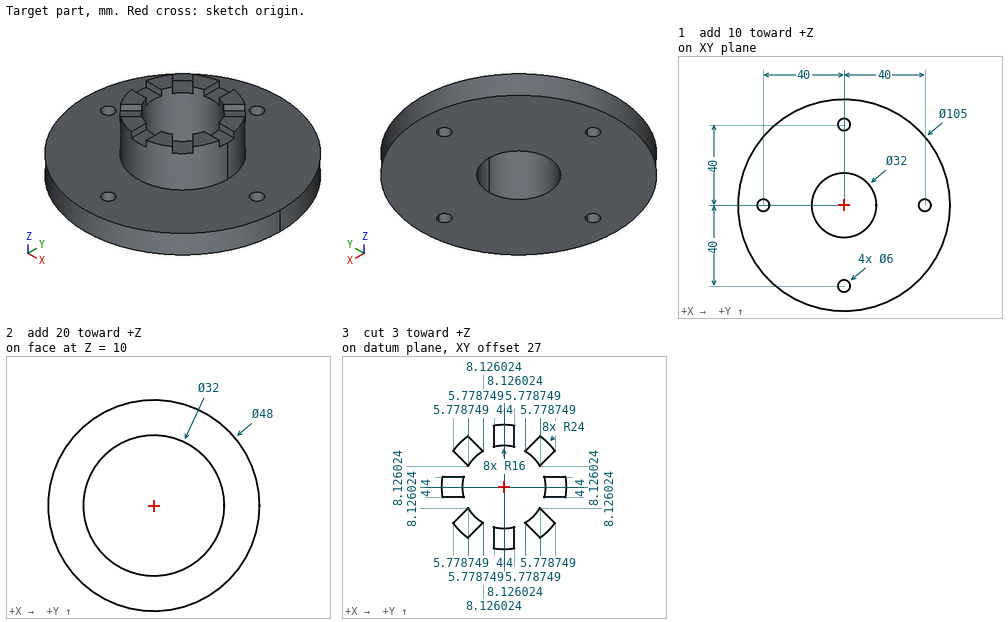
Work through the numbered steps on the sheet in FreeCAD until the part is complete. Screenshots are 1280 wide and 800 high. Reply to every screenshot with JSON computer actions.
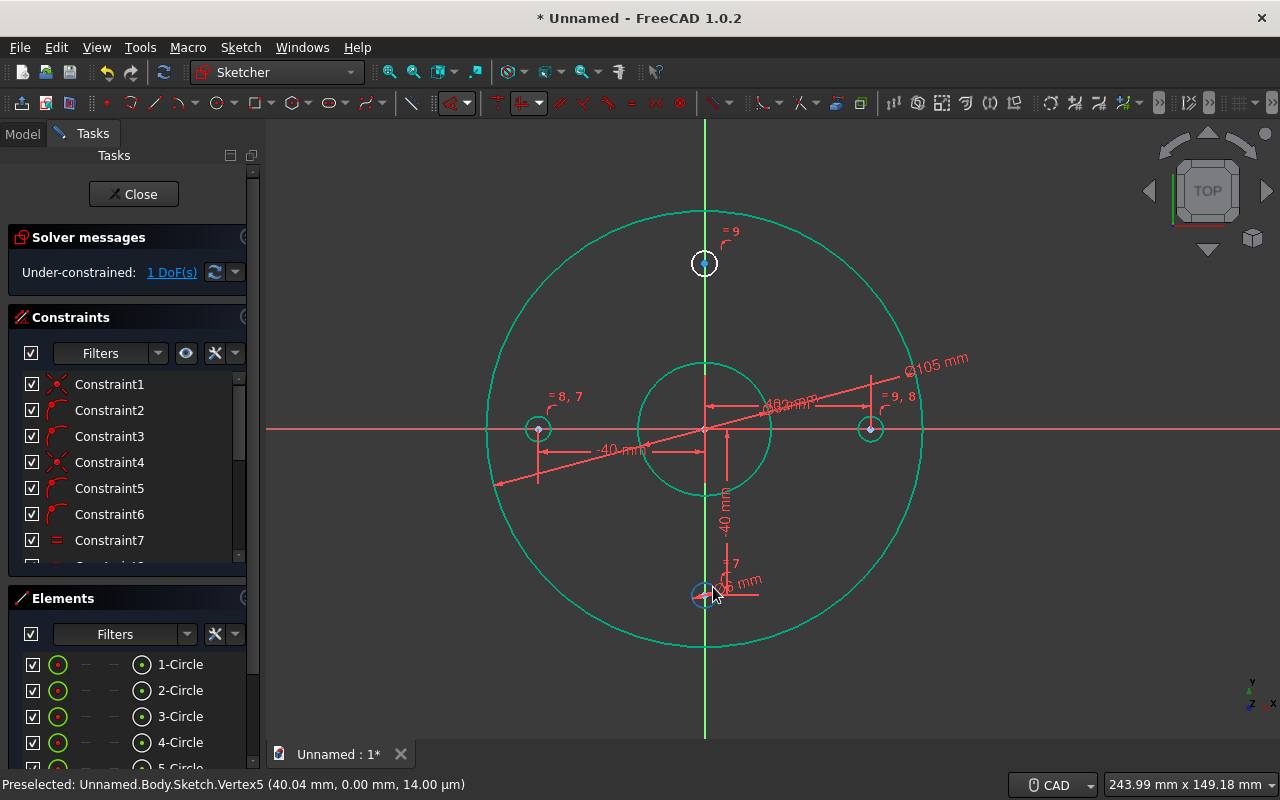
{"action": "left_click", "coordinate": [705, 264]}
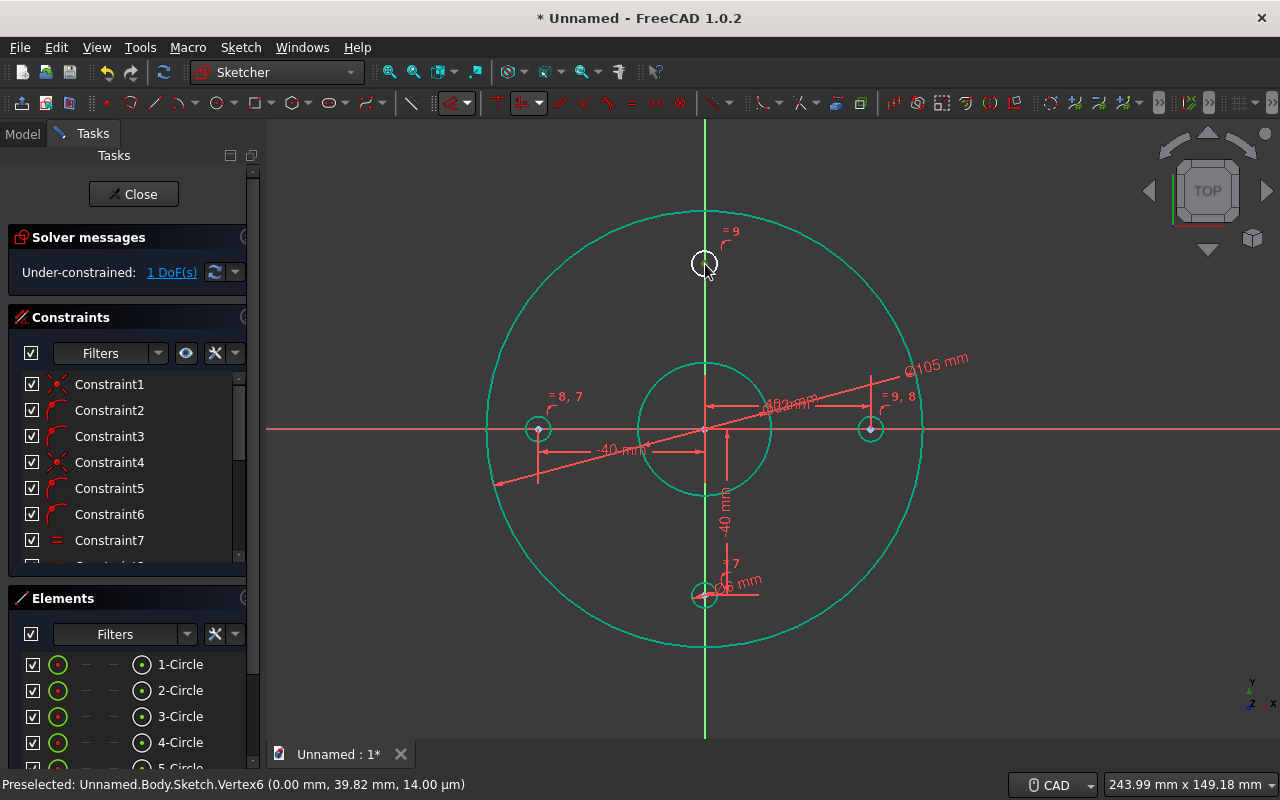
{"action": "key", "text": "i"}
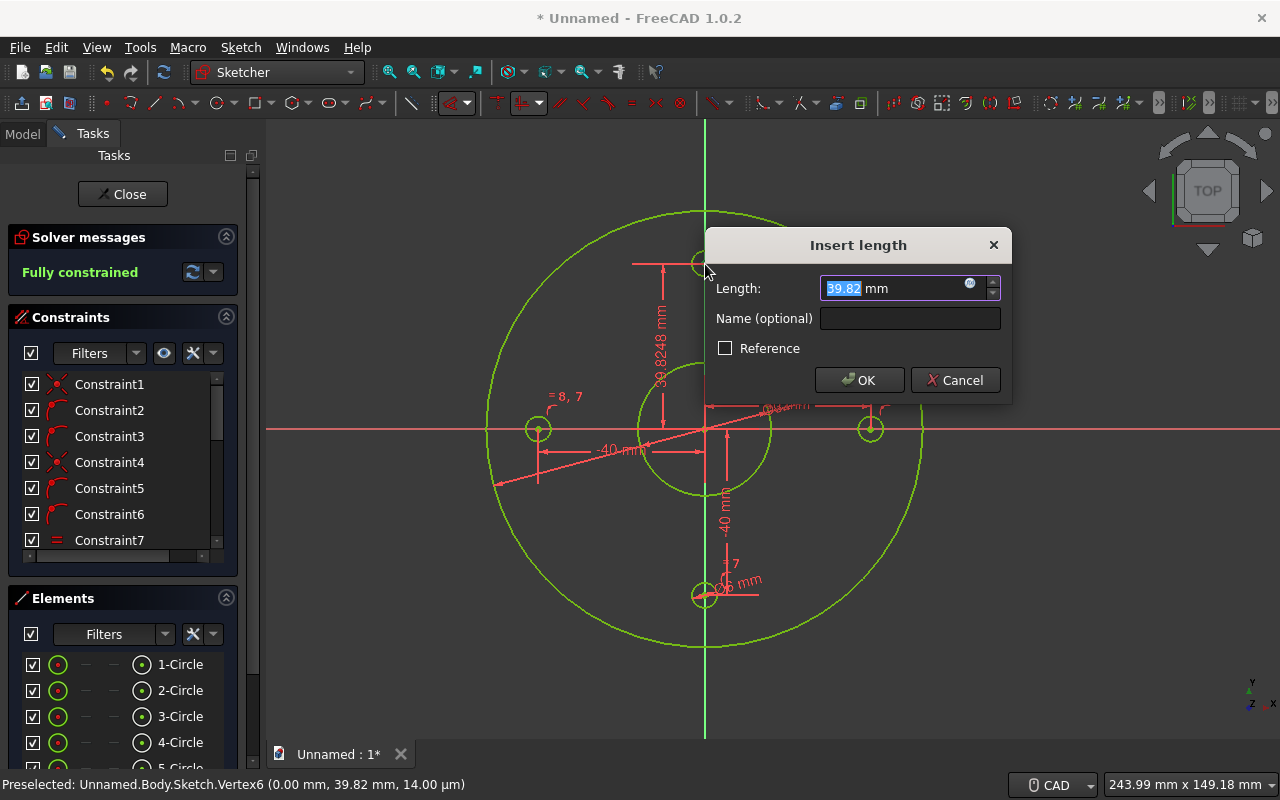
{"action": "type", "text": "40"}
{"action": "key", "text": "Return"}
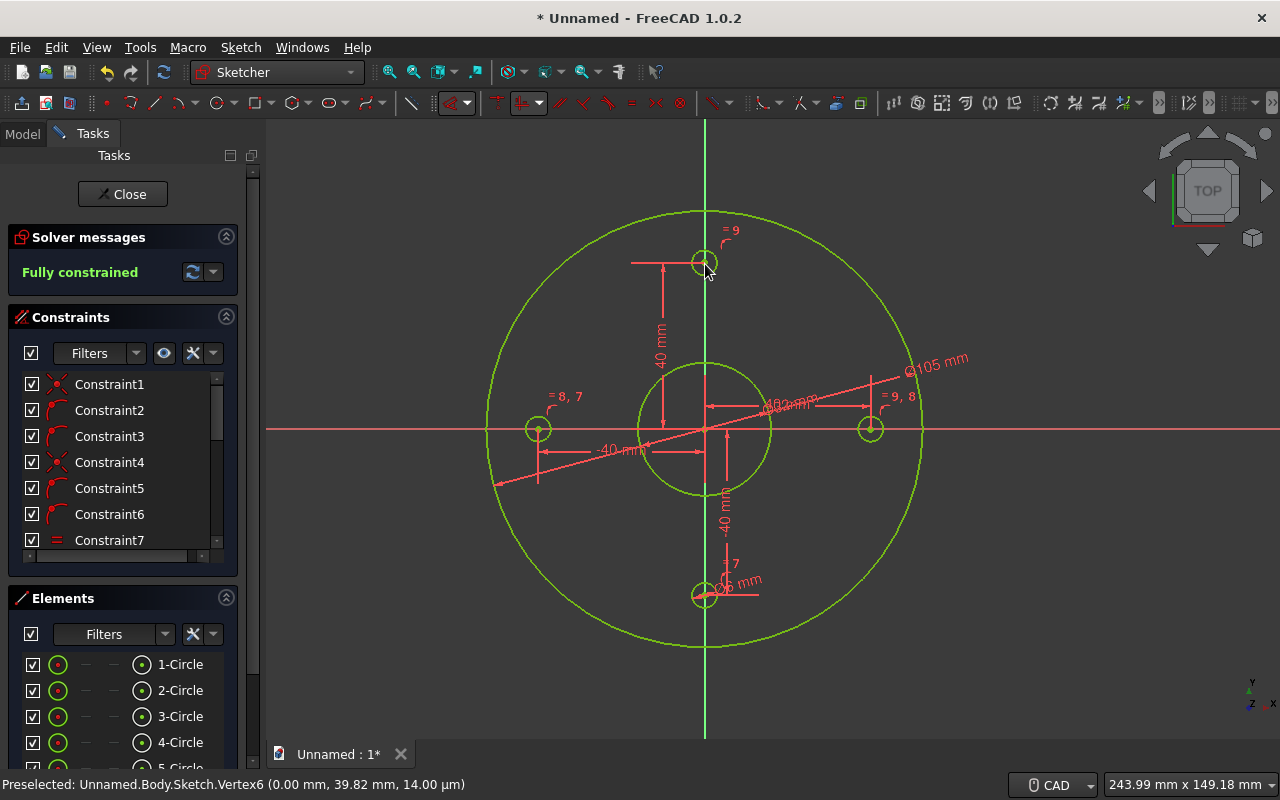
{"action": "left_click", "coordinate": [123, 194]}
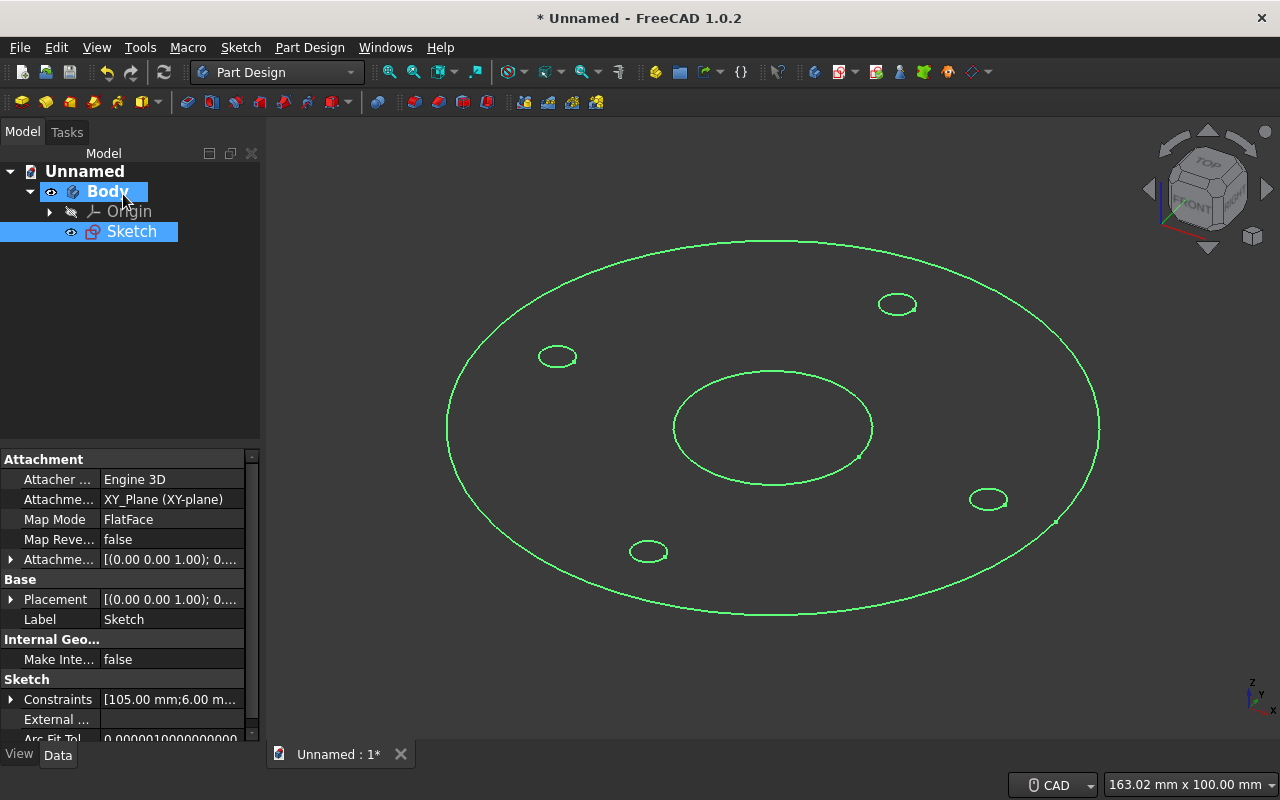
{"action": "left_click", "coordinate": [22, 102]}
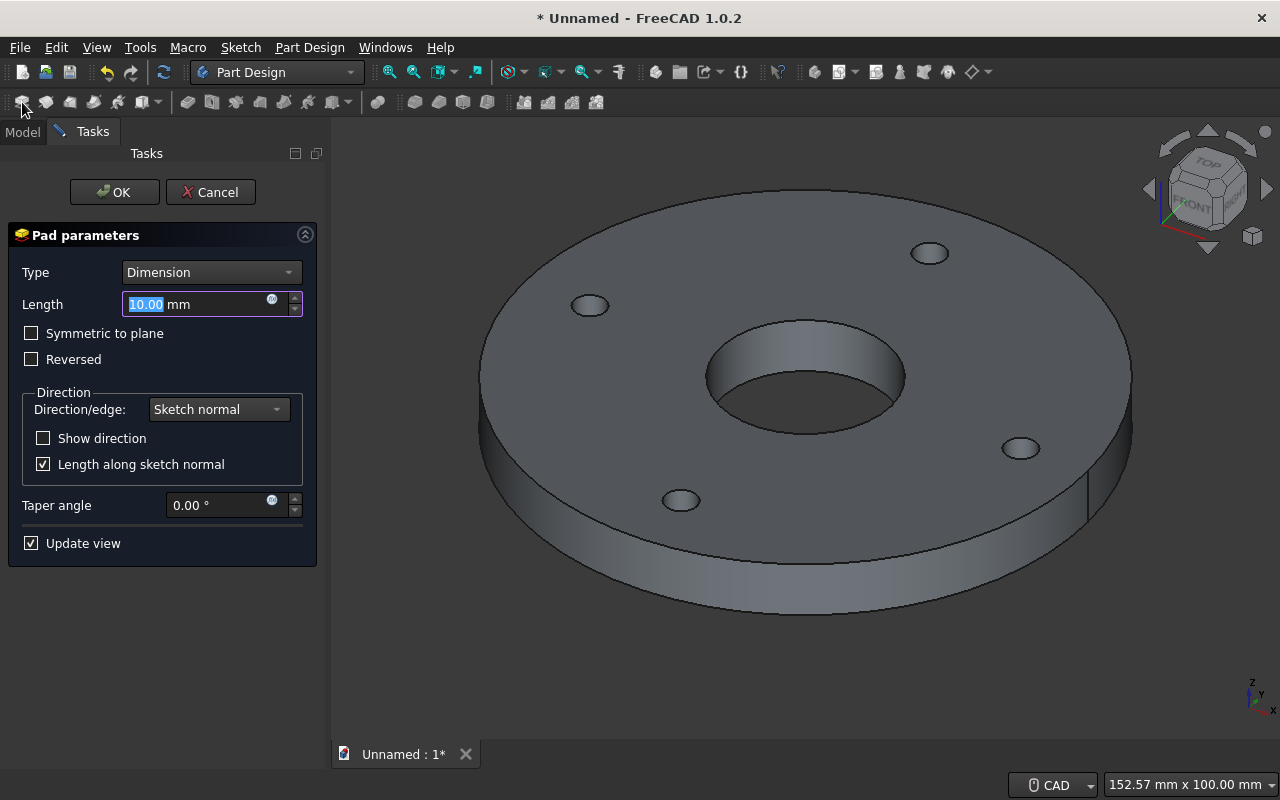
{"action": "type", "text": "10"}
{"action": "key", "text": "Tab"}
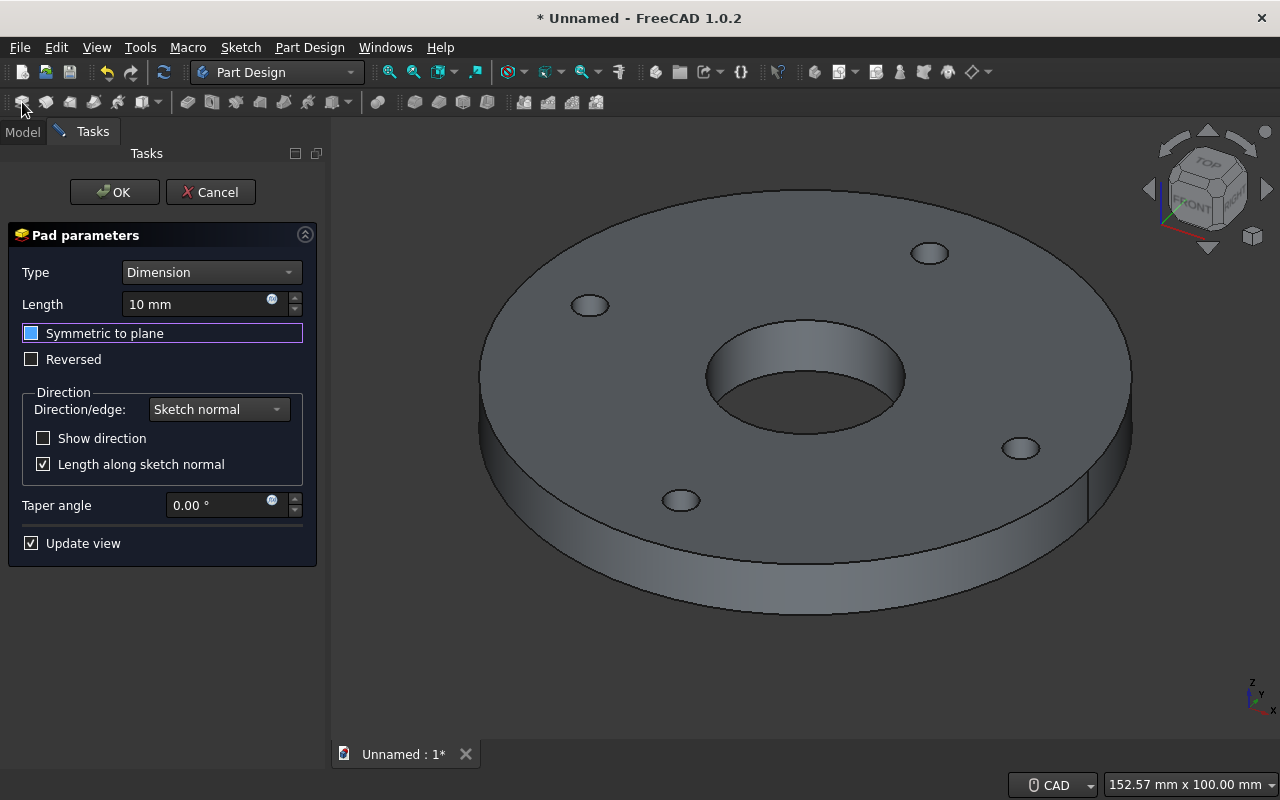
{"action": "left_click", "coordinate": [115, 192]}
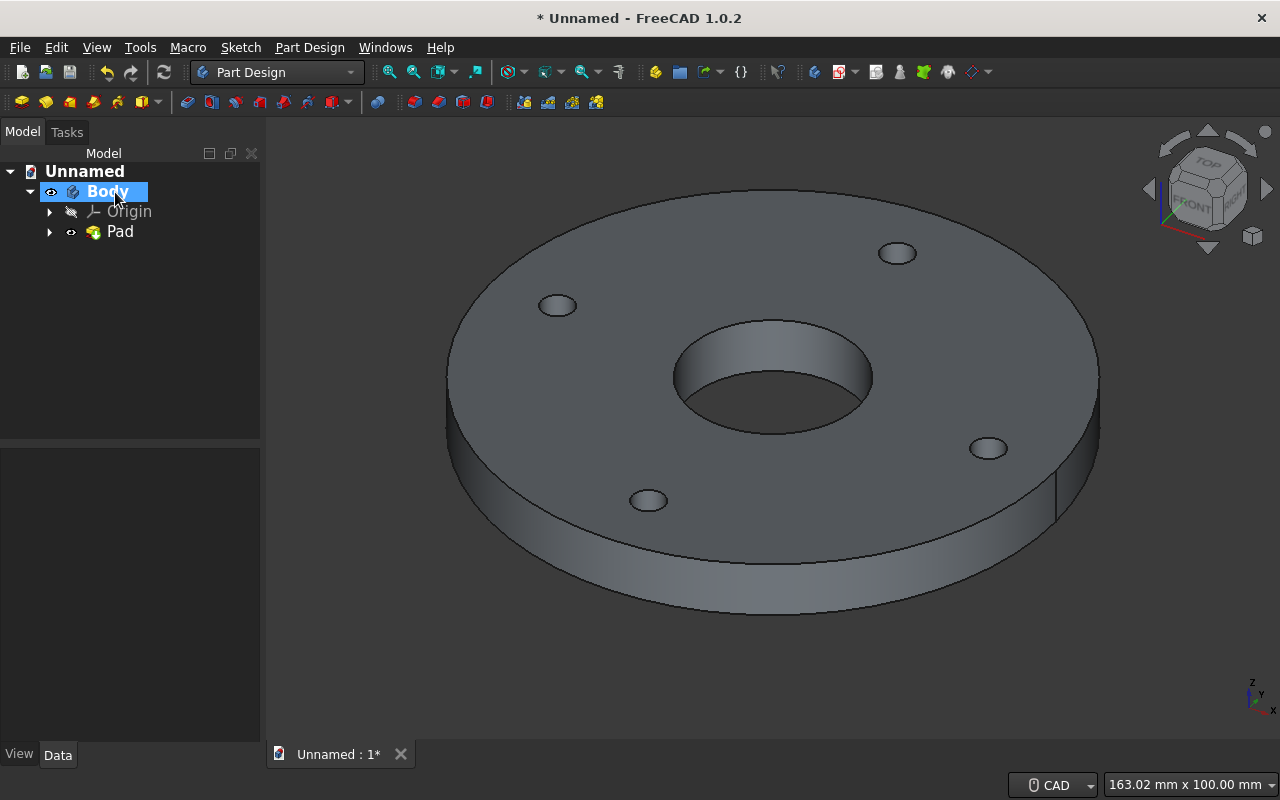
{"action": "left_click", "coordinate": [981, 383]}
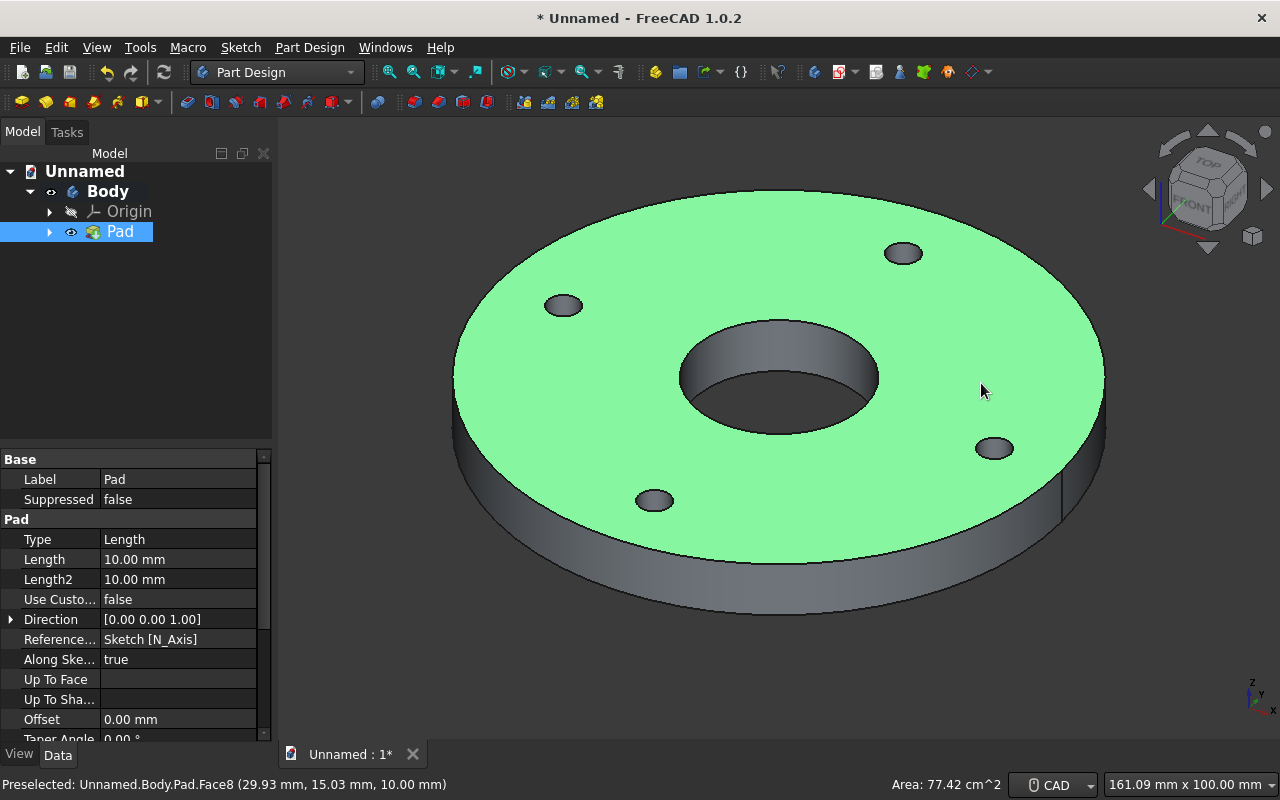
{"action": "left_click", "coordinate": [840, 72]}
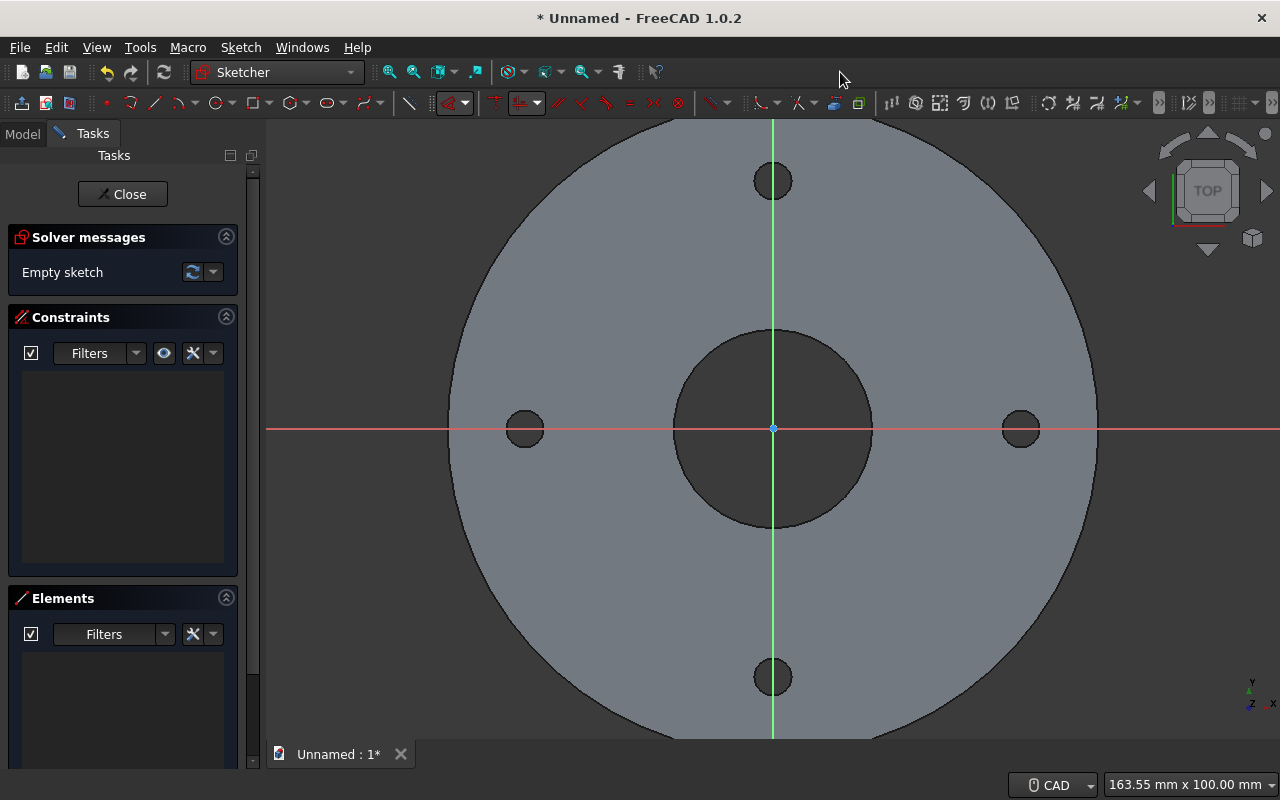
{"action": "left_click", "coordinate": [216, 104]}